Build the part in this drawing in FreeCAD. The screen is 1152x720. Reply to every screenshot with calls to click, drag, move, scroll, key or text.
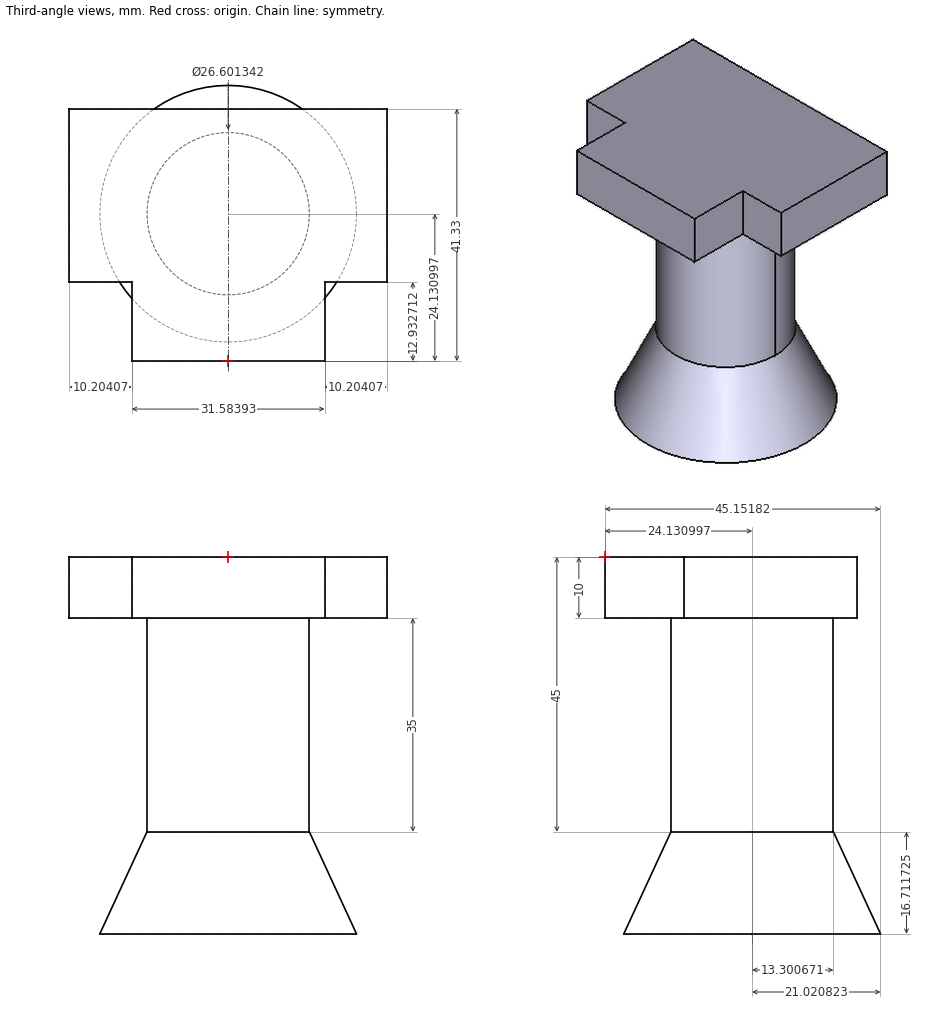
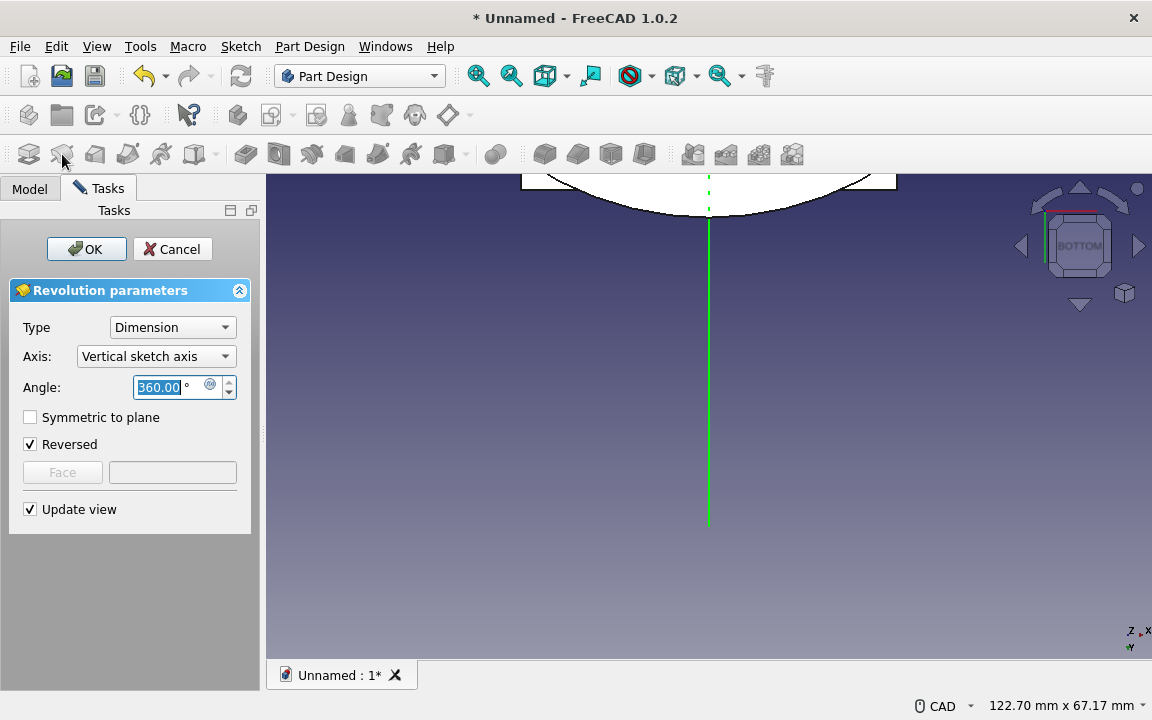
click(157, 356)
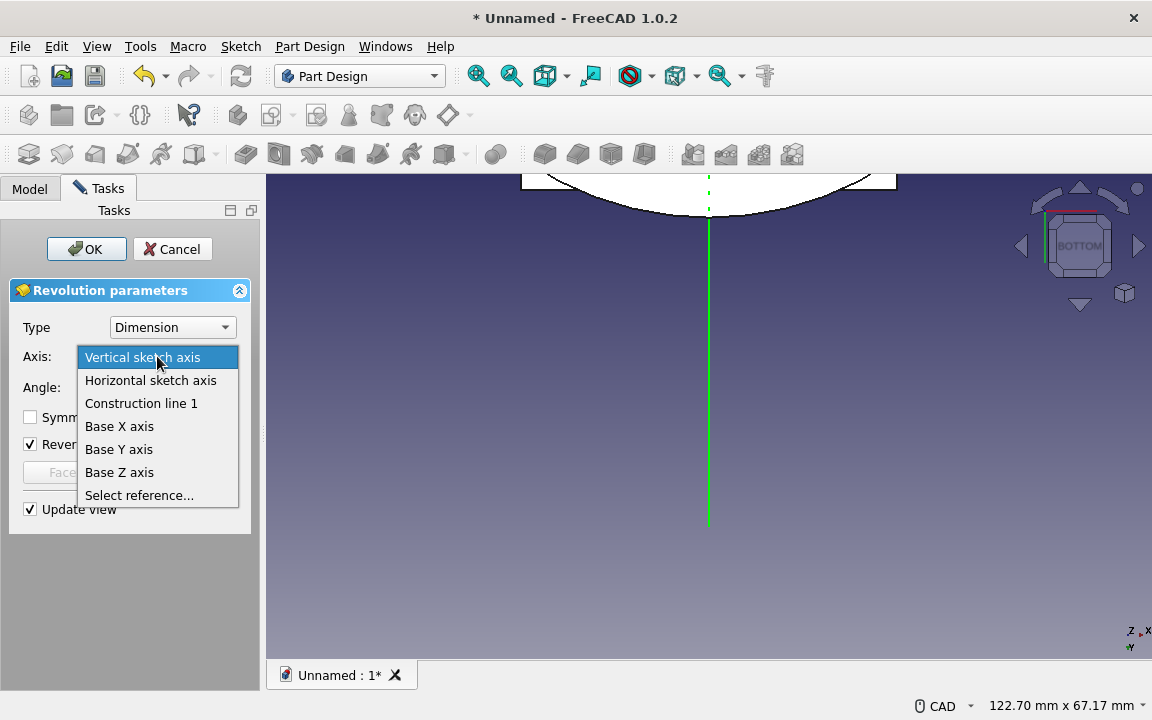
click(156, 404)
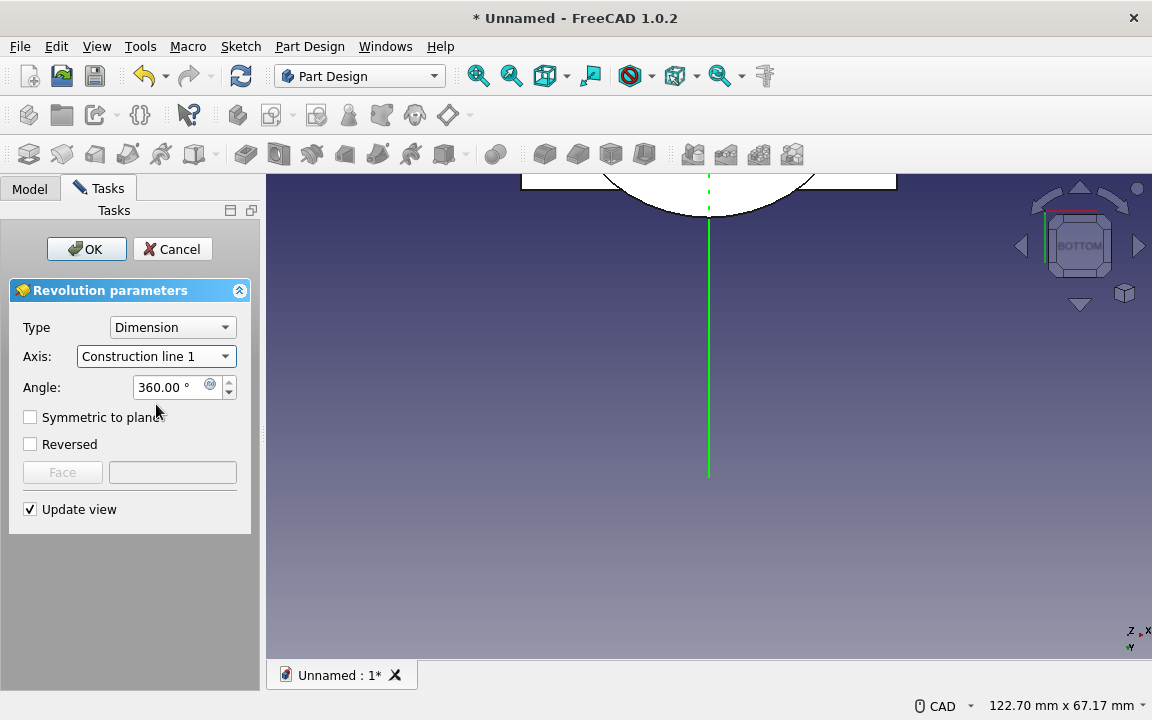
click(87, 249)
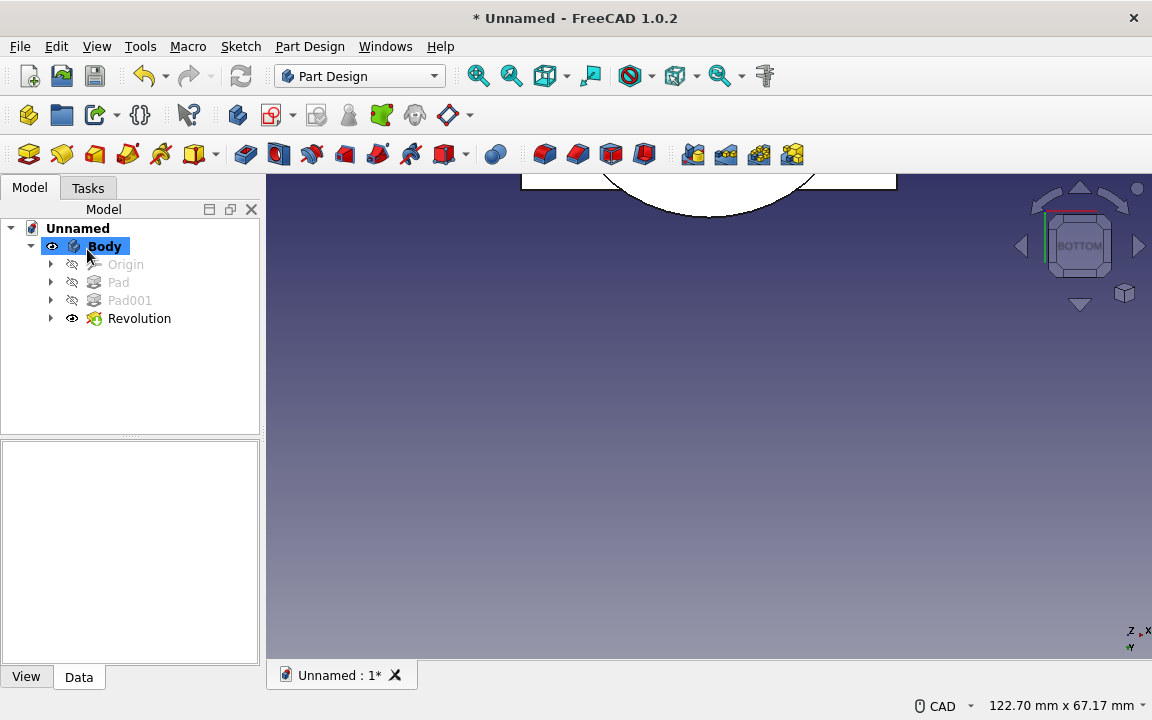
key(0)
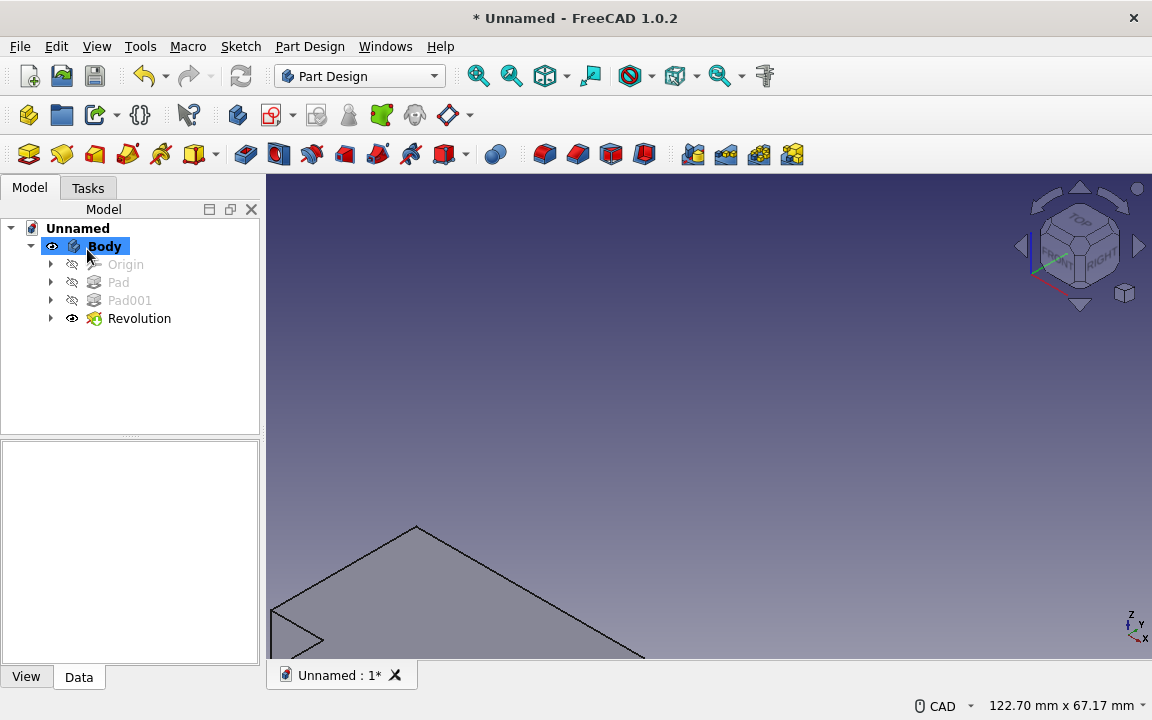
click(479, 76)